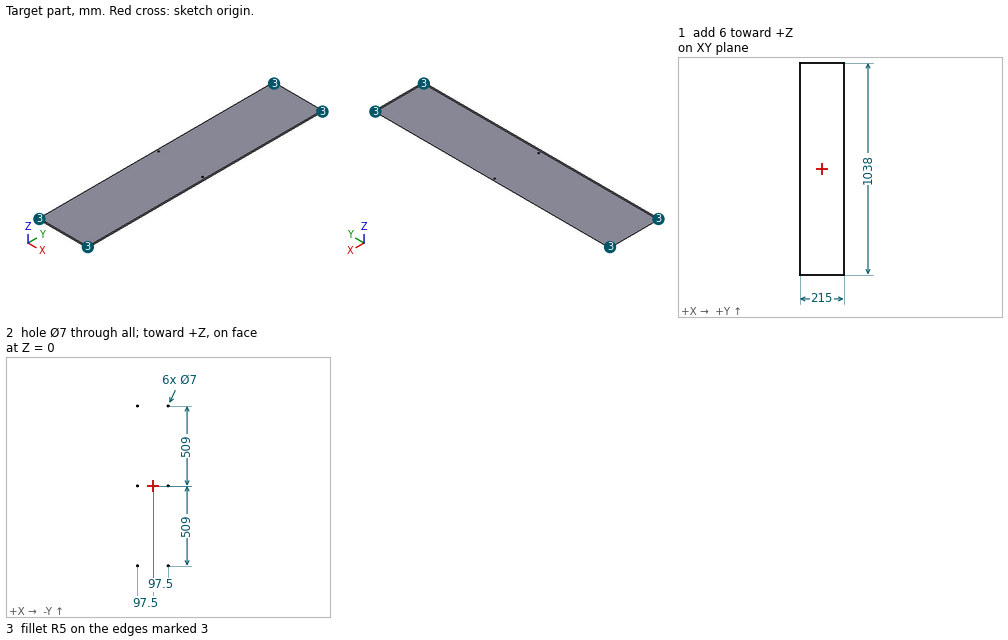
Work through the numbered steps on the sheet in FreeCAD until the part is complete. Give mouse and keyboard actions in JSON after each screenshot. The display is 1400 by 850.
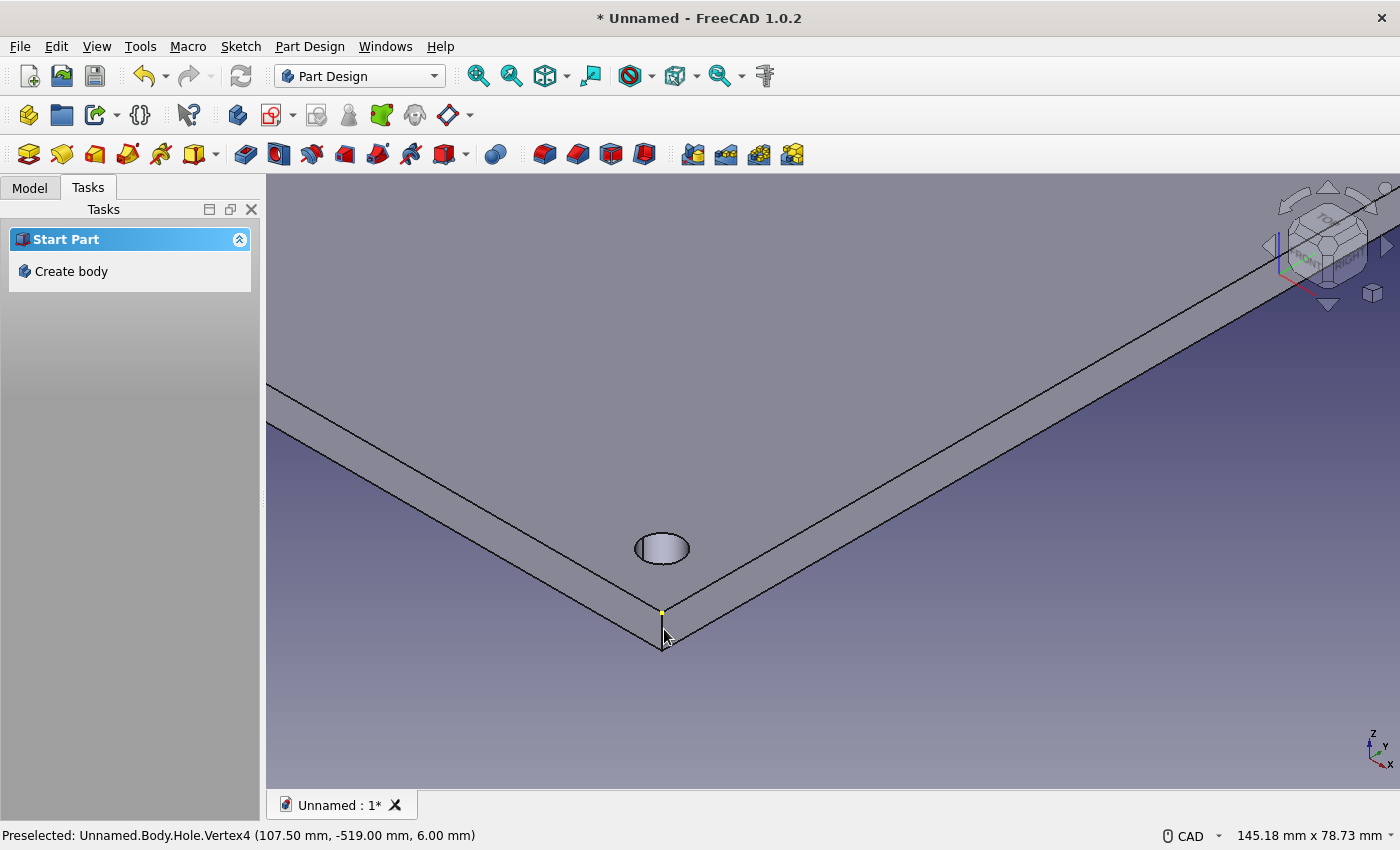
{"action": "left_click", "coordinate": [662, 631]}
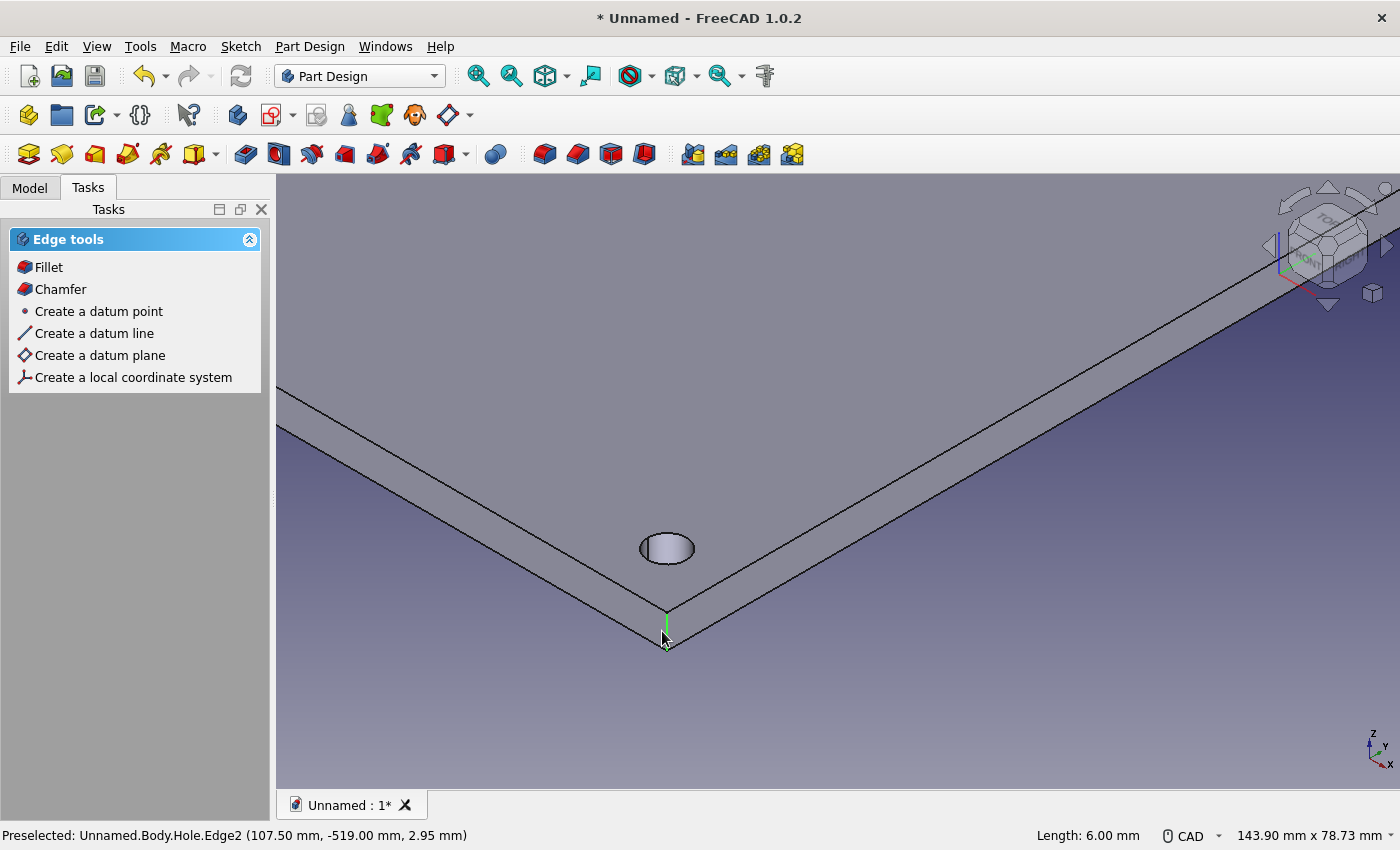
{"action": "left_click", "coordinate": [479, 76]}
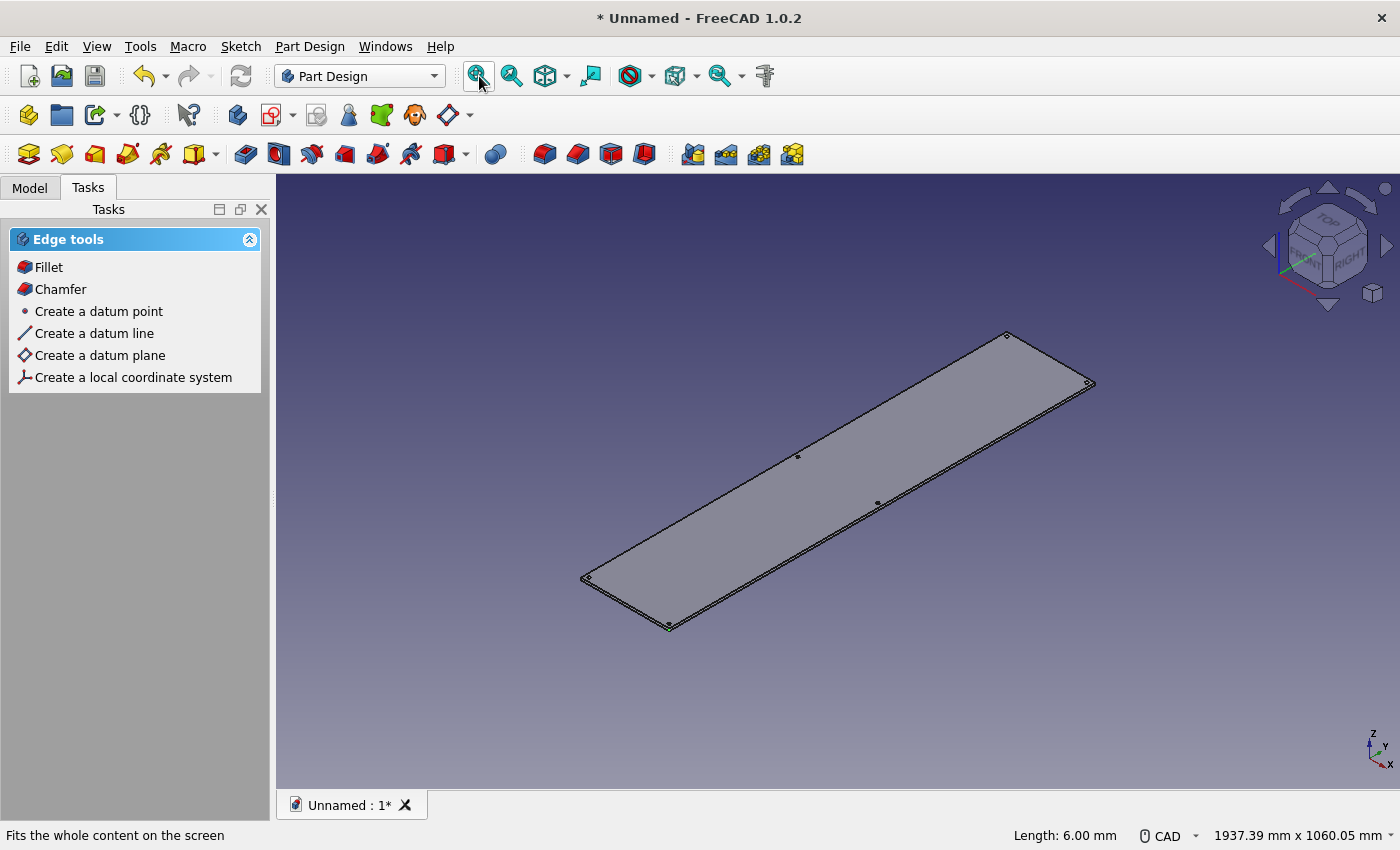
{"action": "key", "text": "2"}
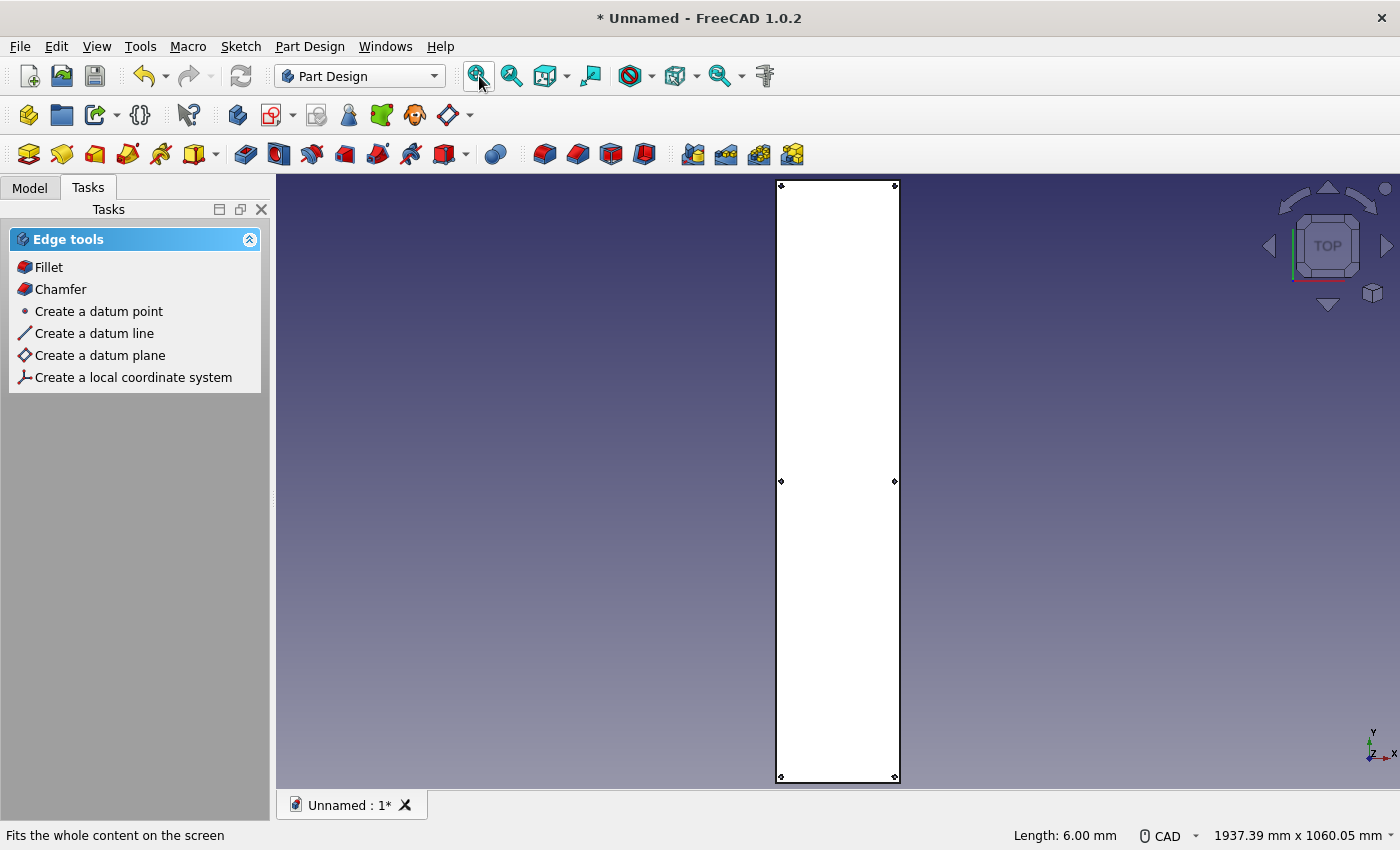
{"action": "key", "text": "1"}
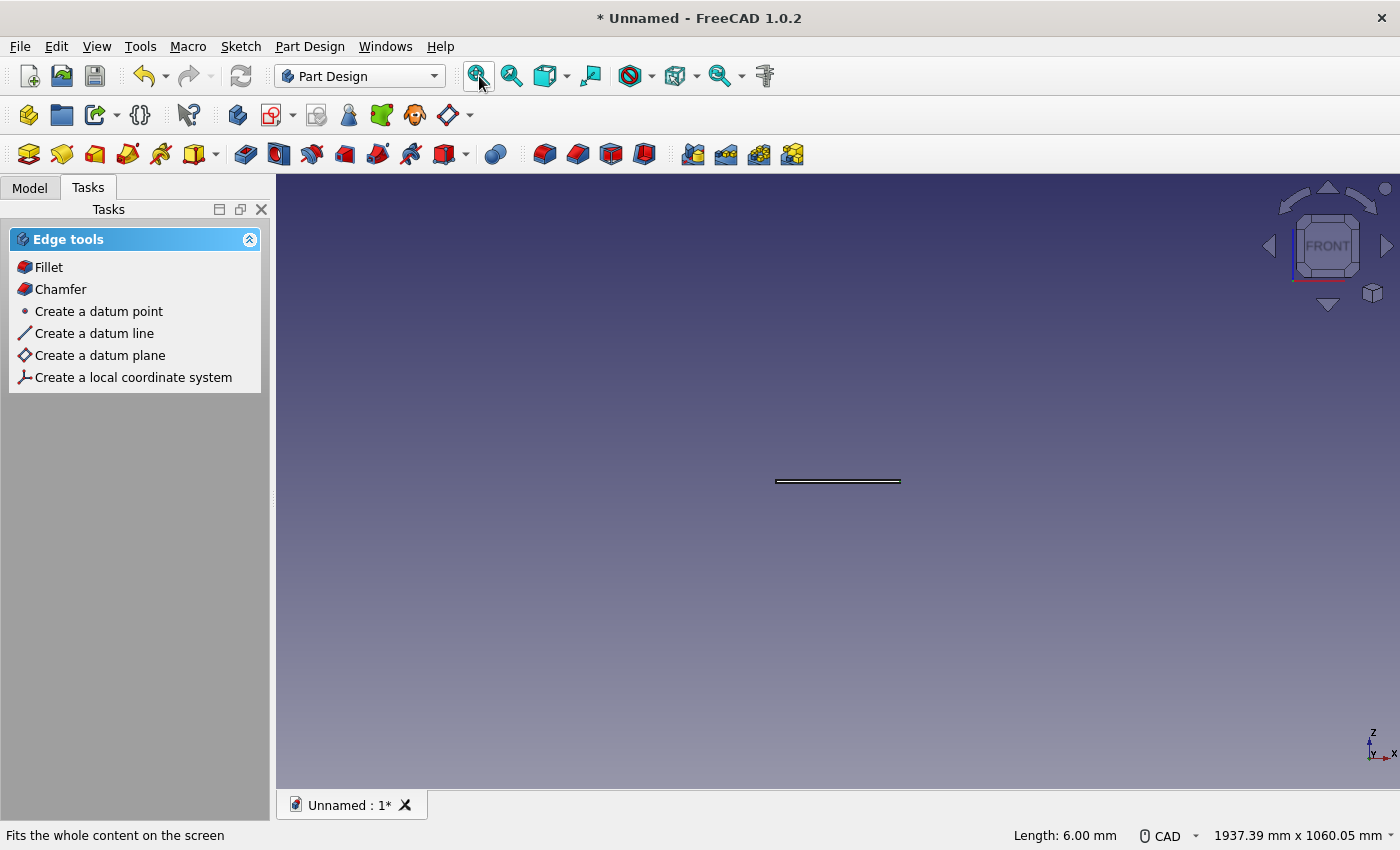
{"action": "left_click", "coordinate": [479, 76]}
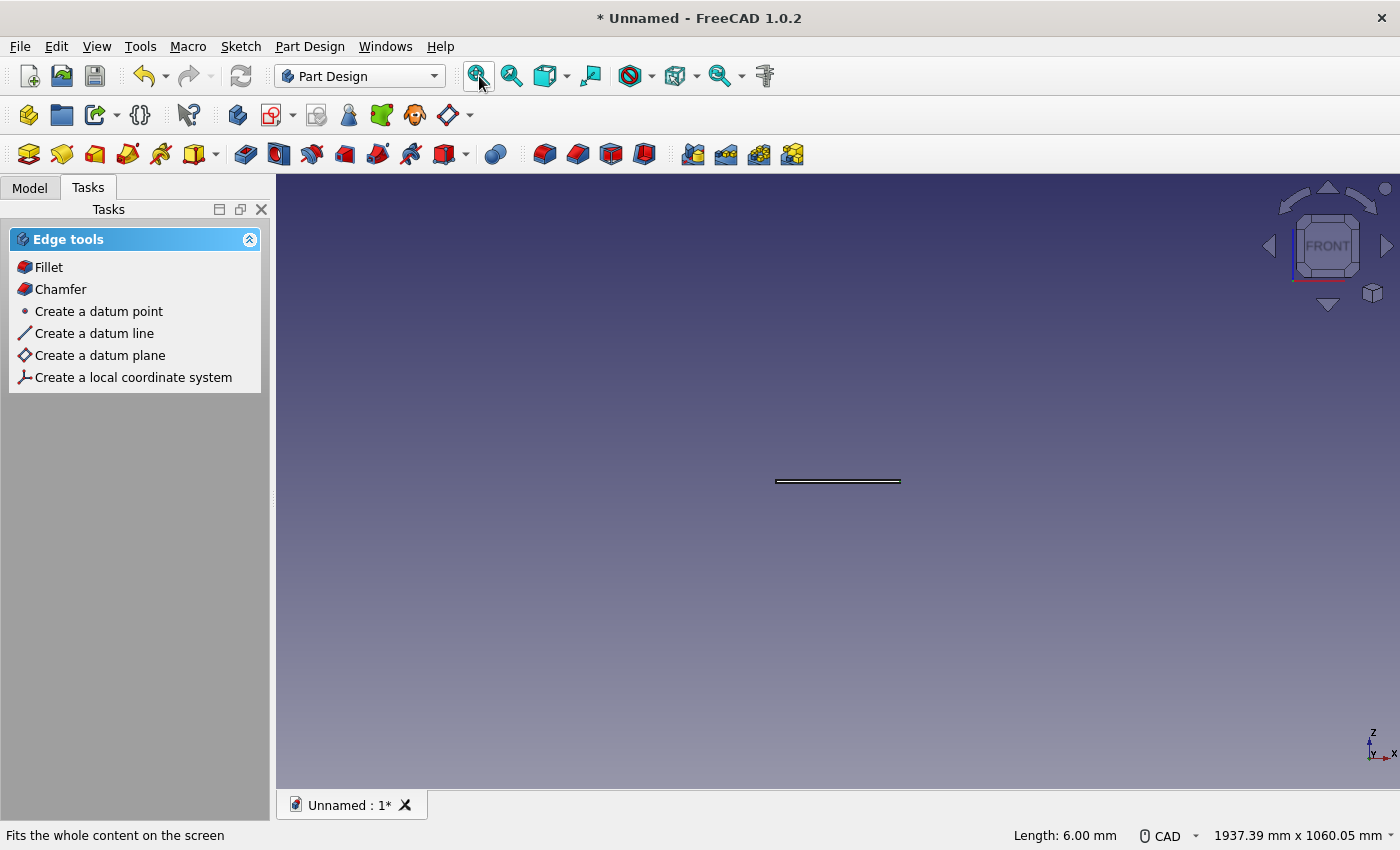
{"action": "scroll", "coordinate": [776, 481], "scroll_direction": "up", "scroll_amount": 13}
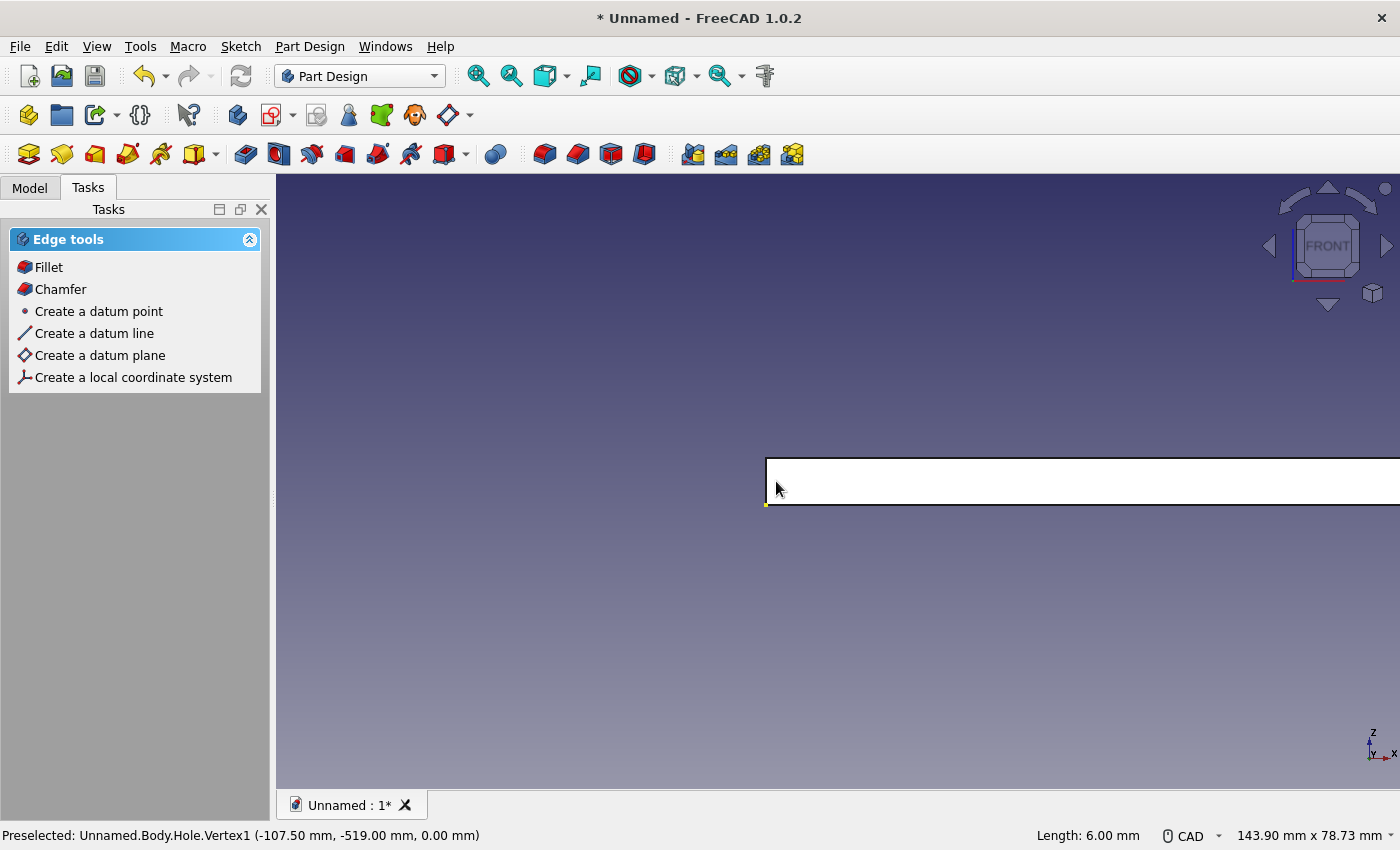
{"action": "left_click", "coordinate": [766, 481], "text": "ctrl"}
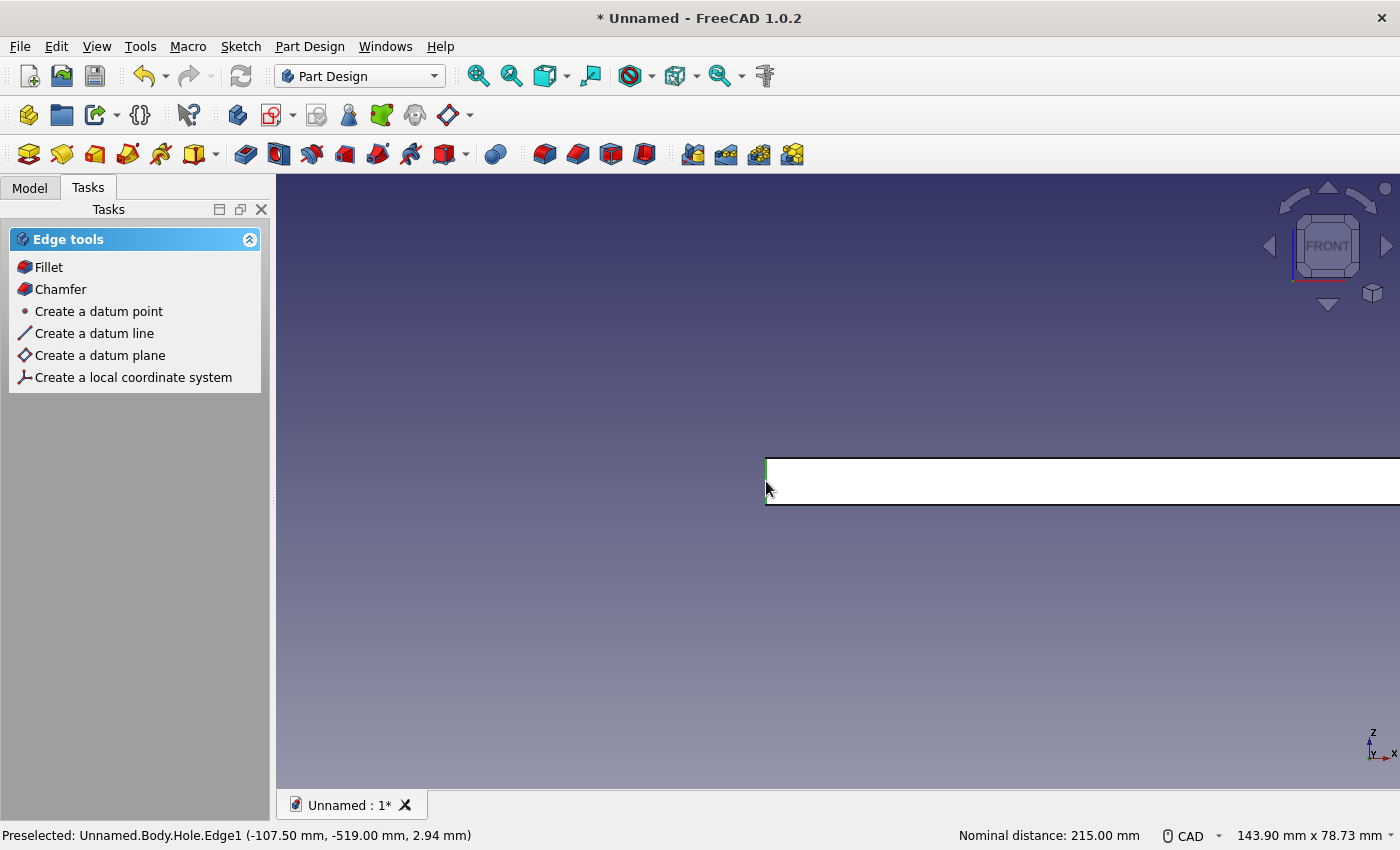
{"action": "key", "text": "v f"}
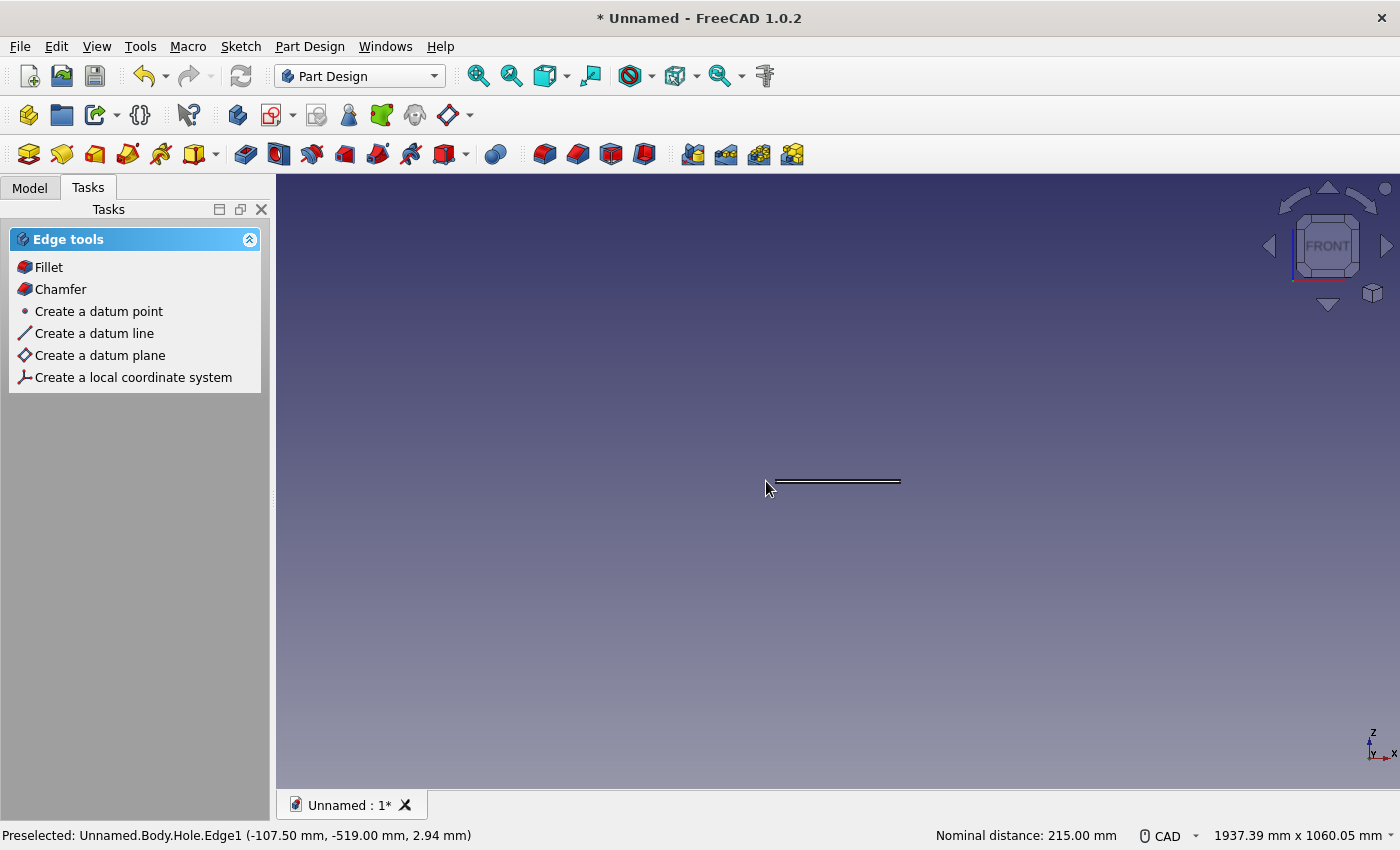
{"action": "key", "text": "3"}